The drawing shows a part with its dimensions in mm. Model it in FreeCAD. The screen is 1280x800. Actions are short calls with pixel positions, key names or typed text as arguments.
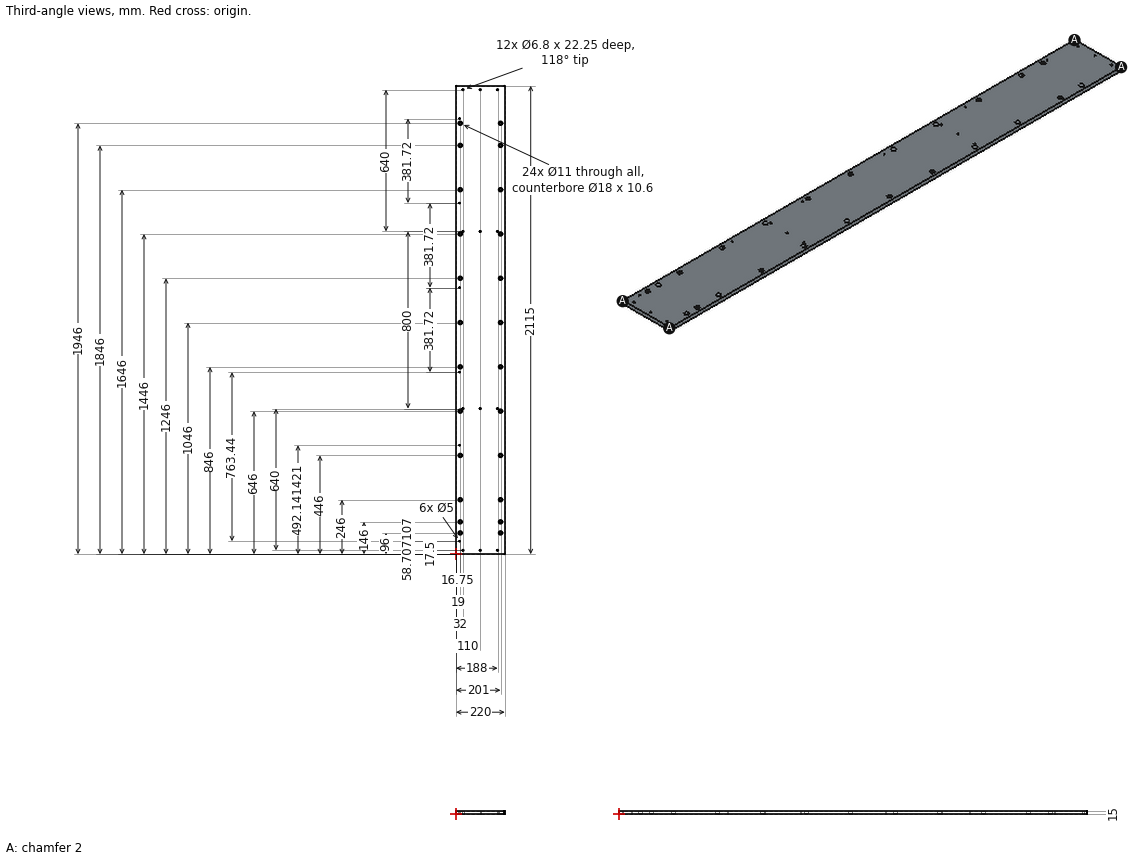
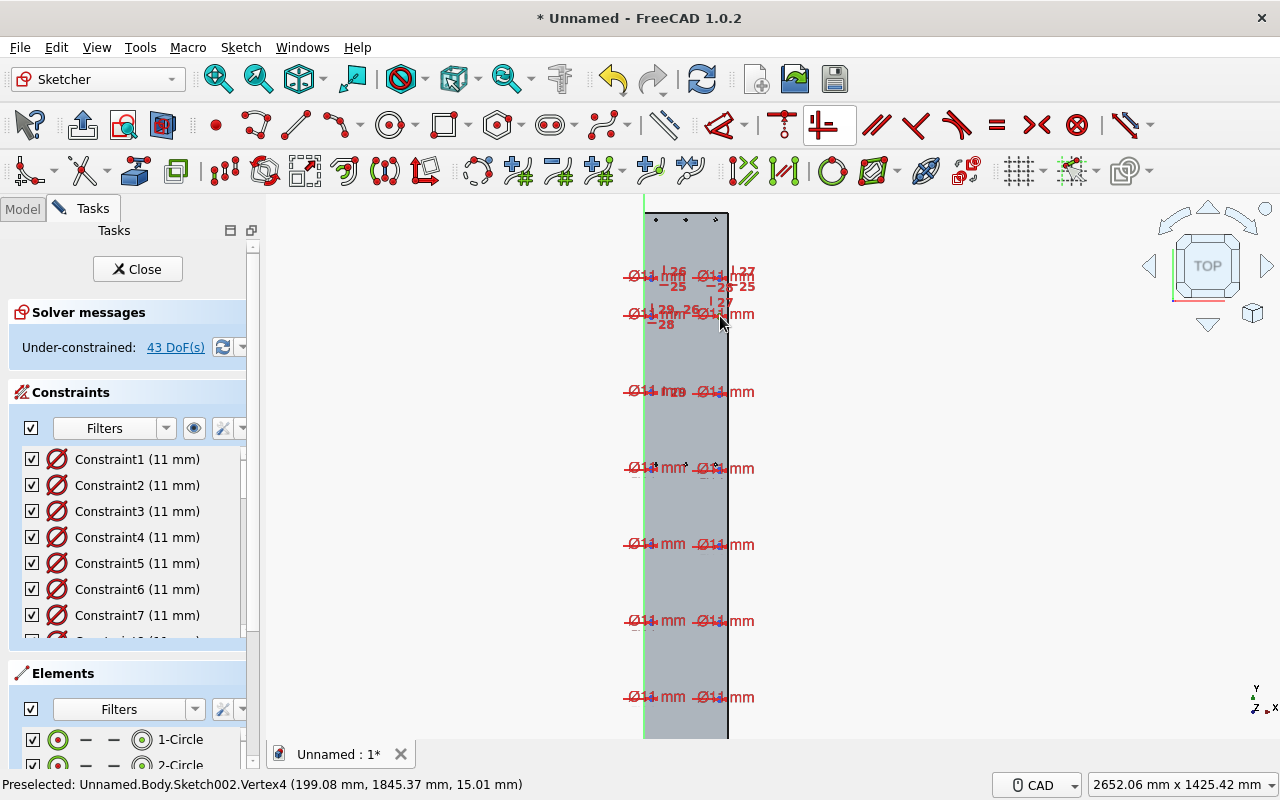
click(720, 394)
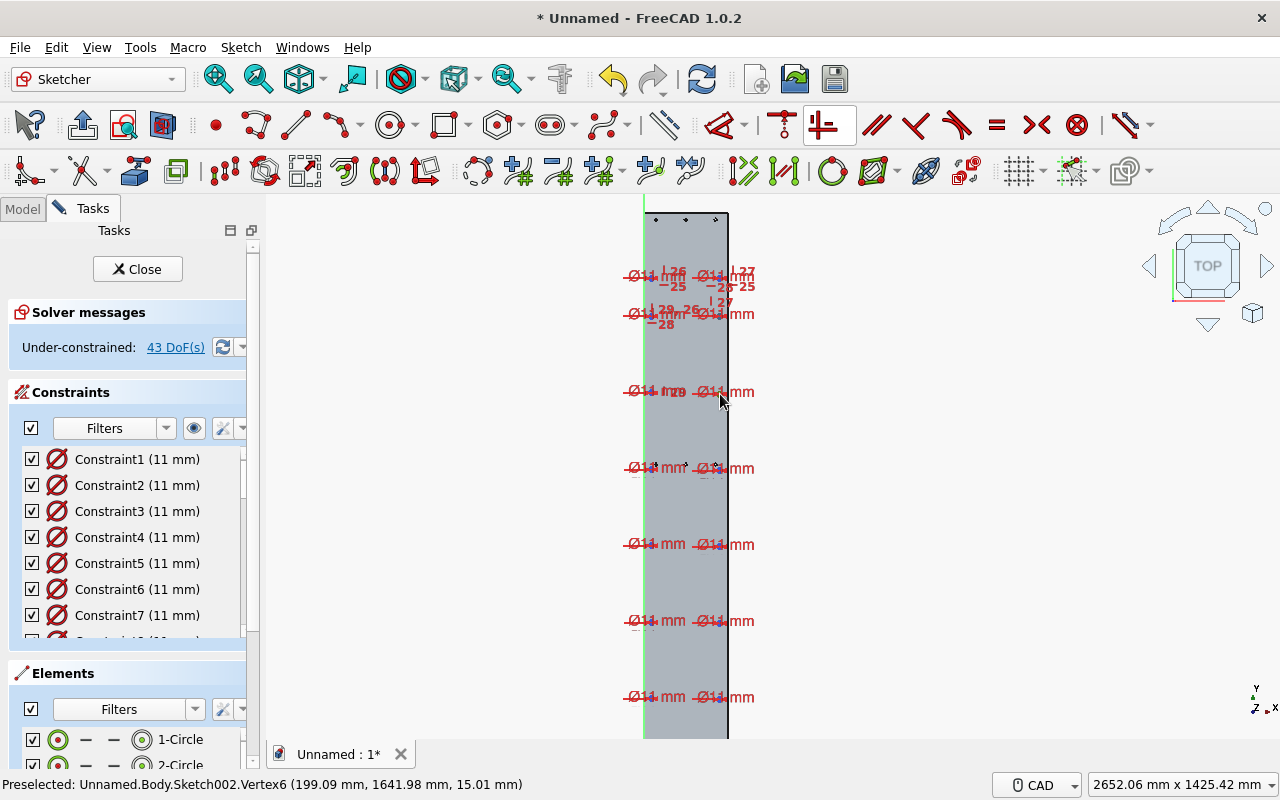
key(v)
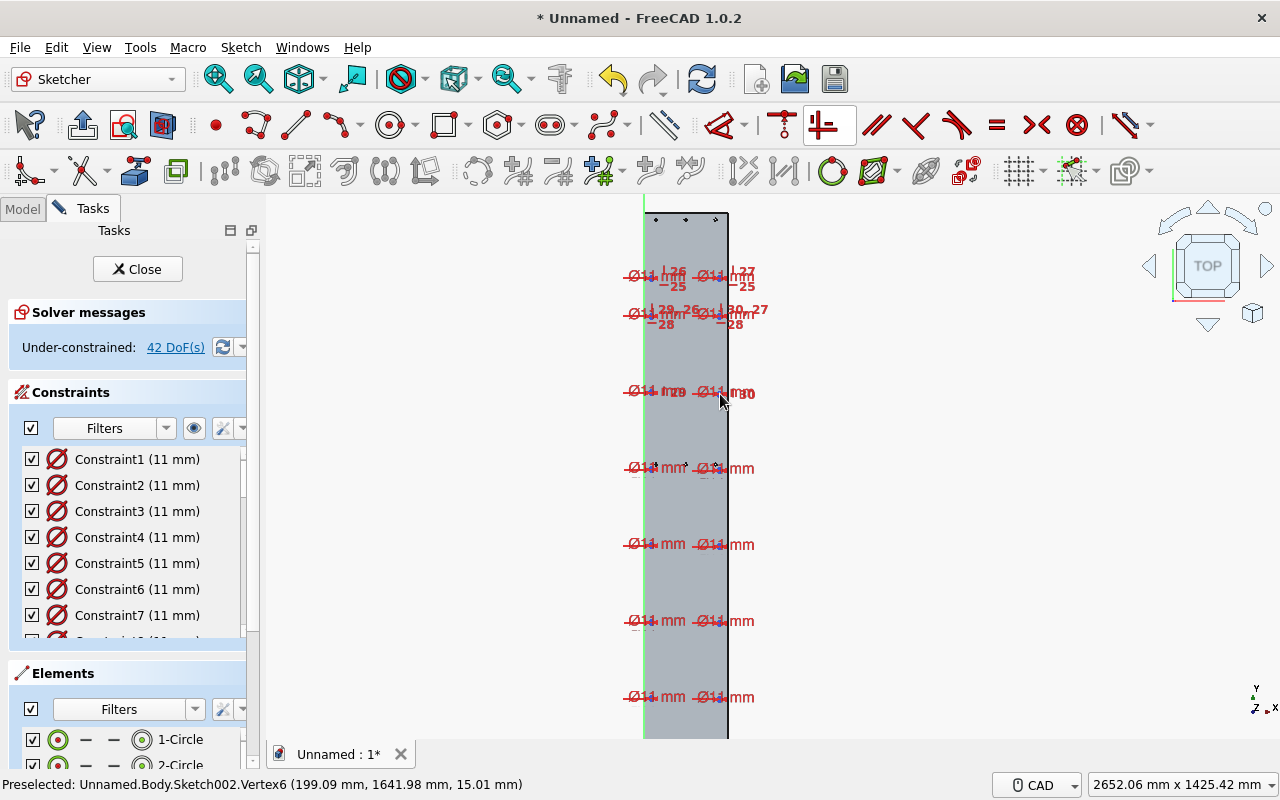
click(651, 393)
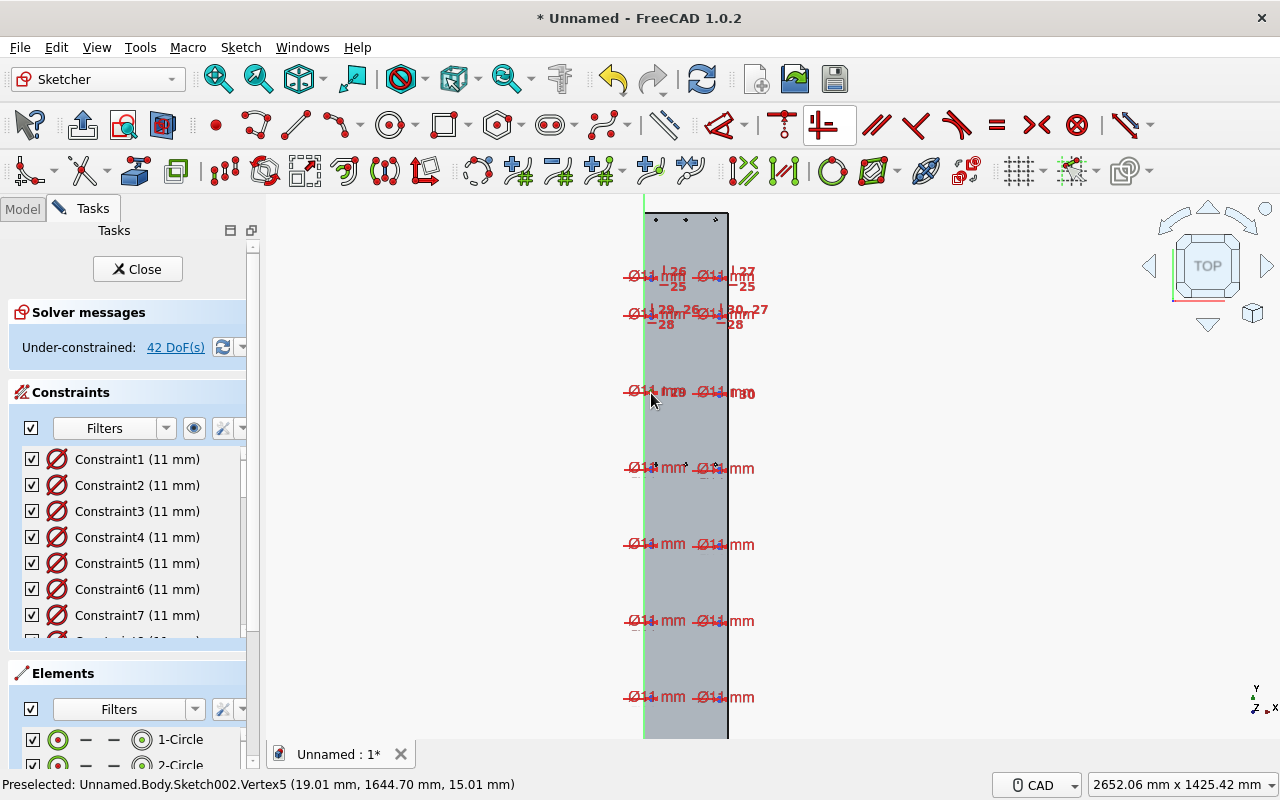
click(720, 394)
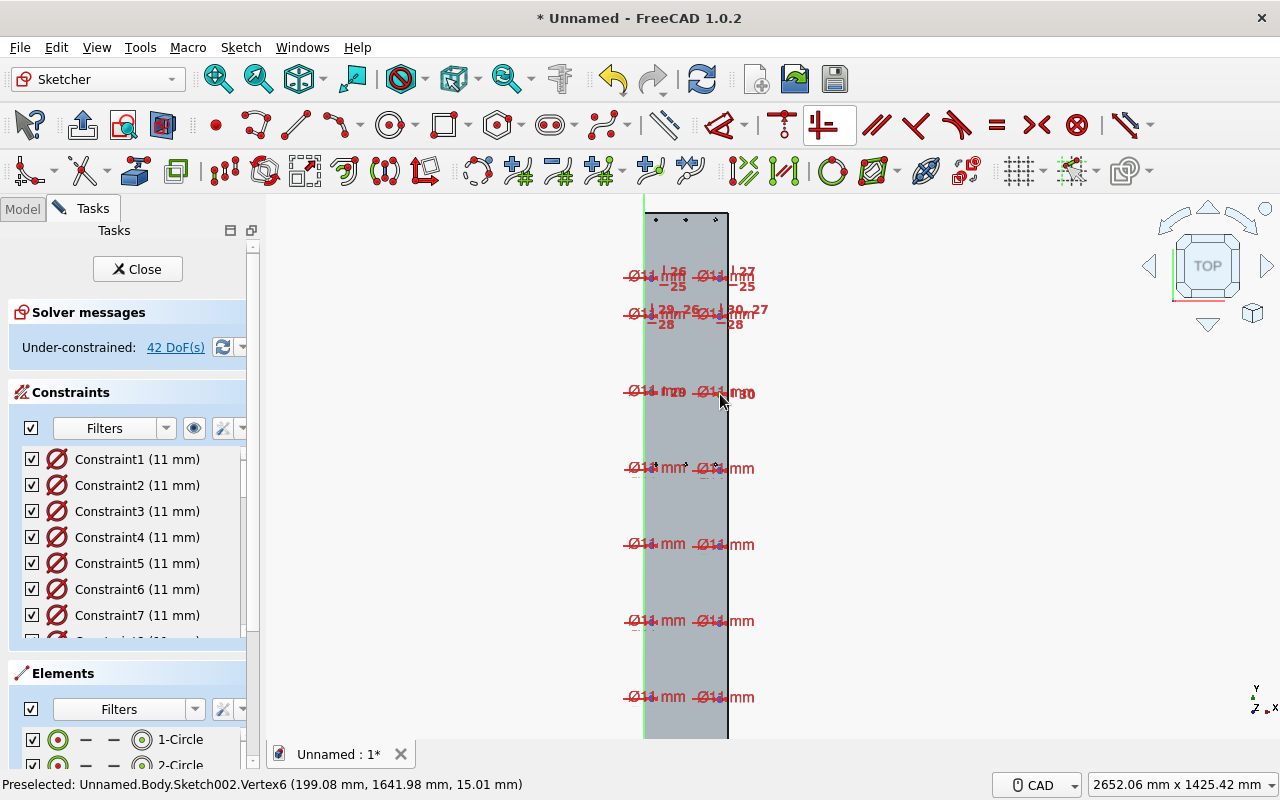
click(850, 126)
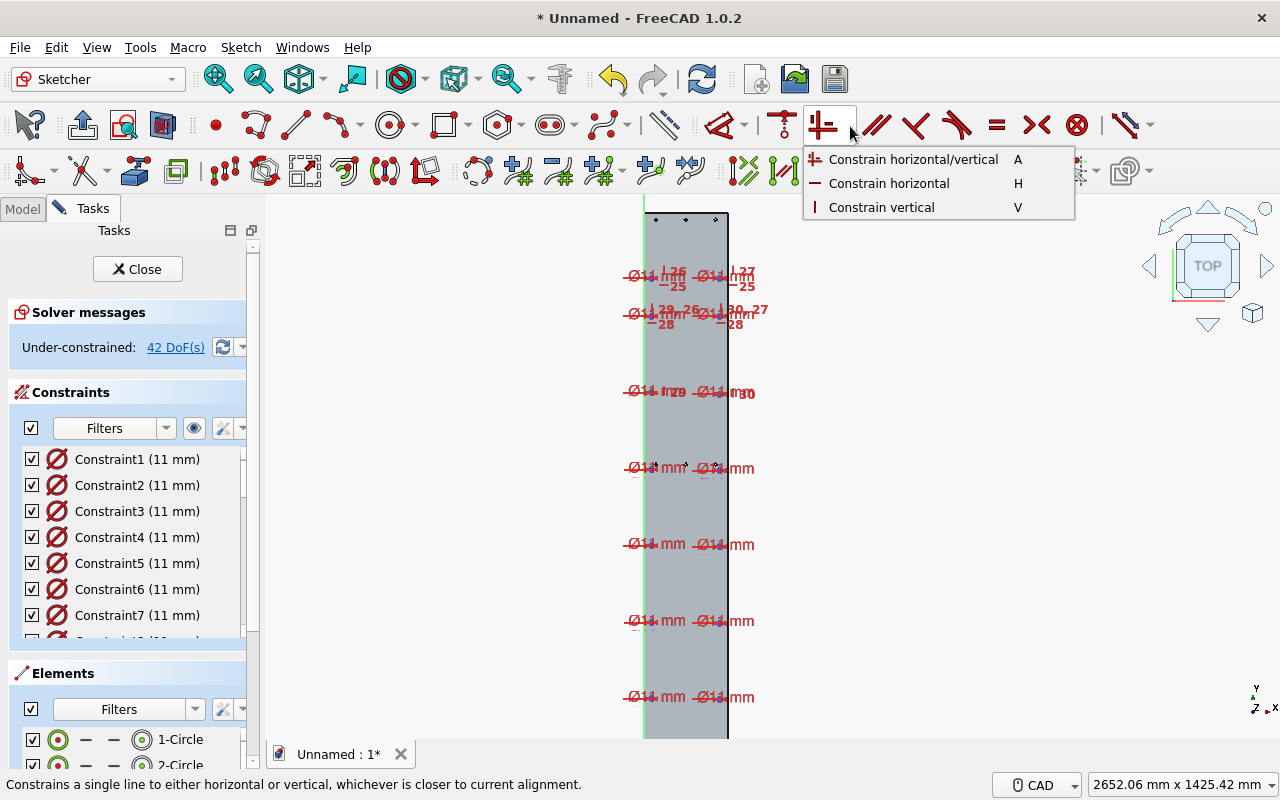
click(939, 183)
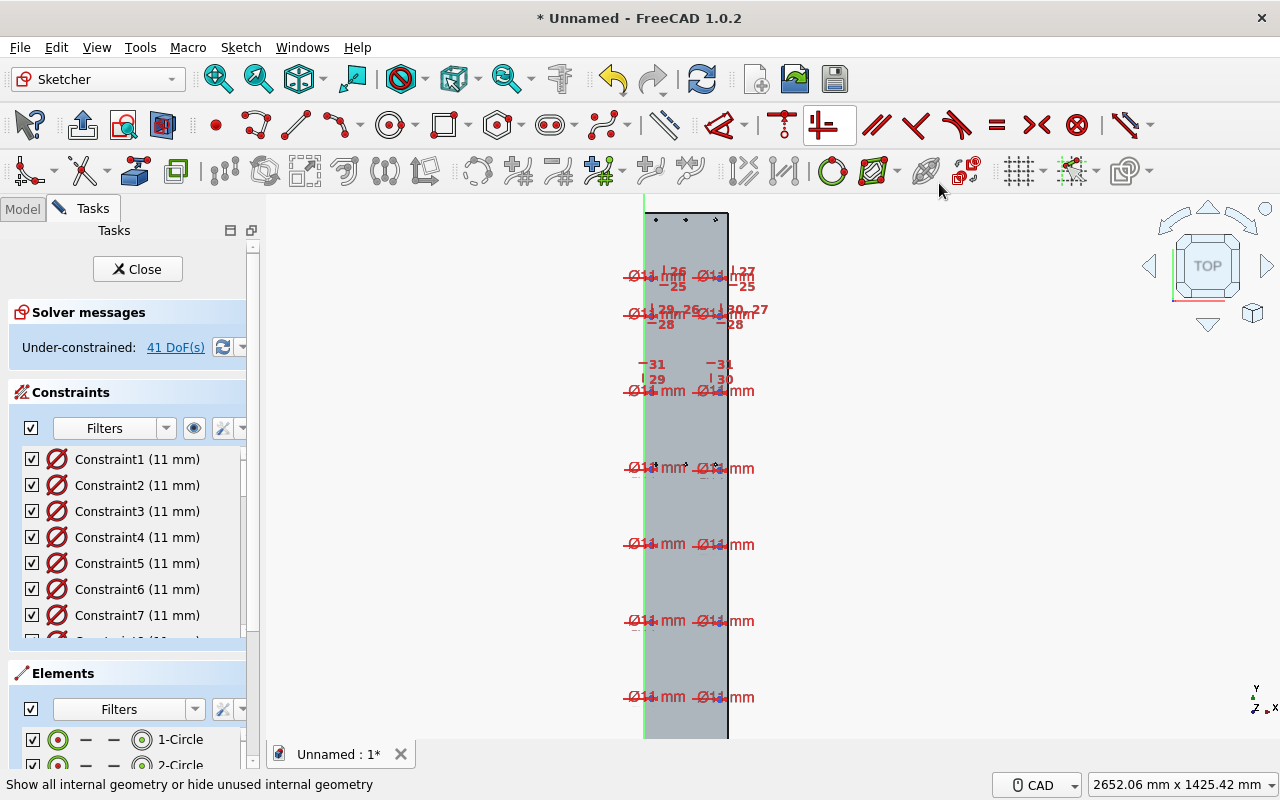
click(651, 393)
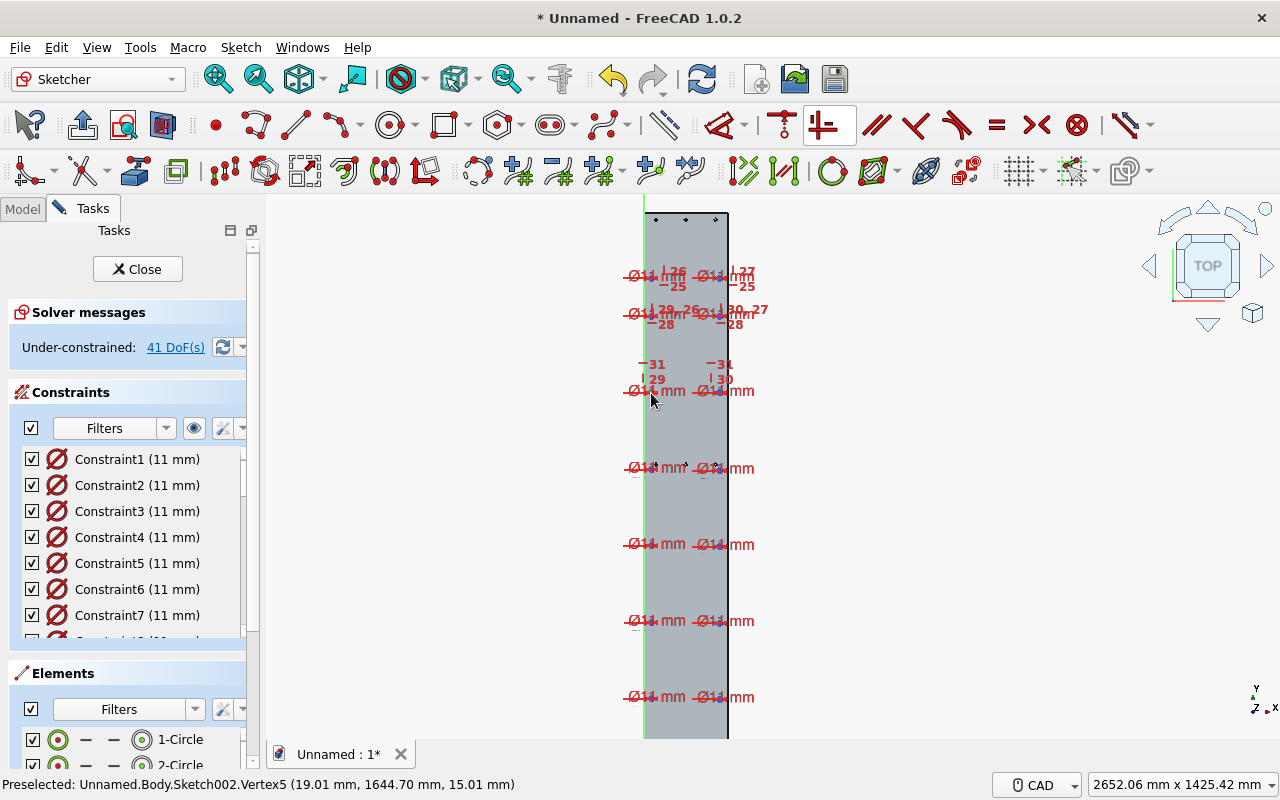
click(651, 470)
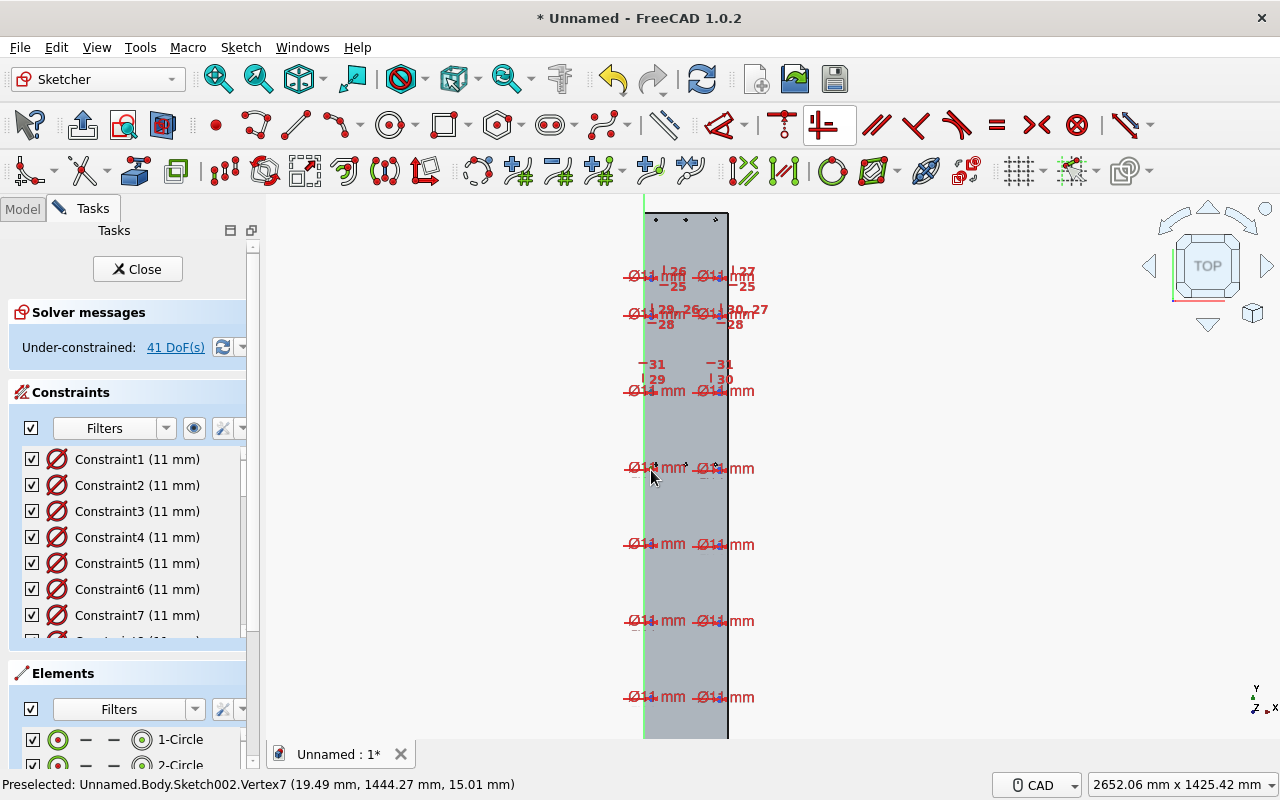
click(850, 126)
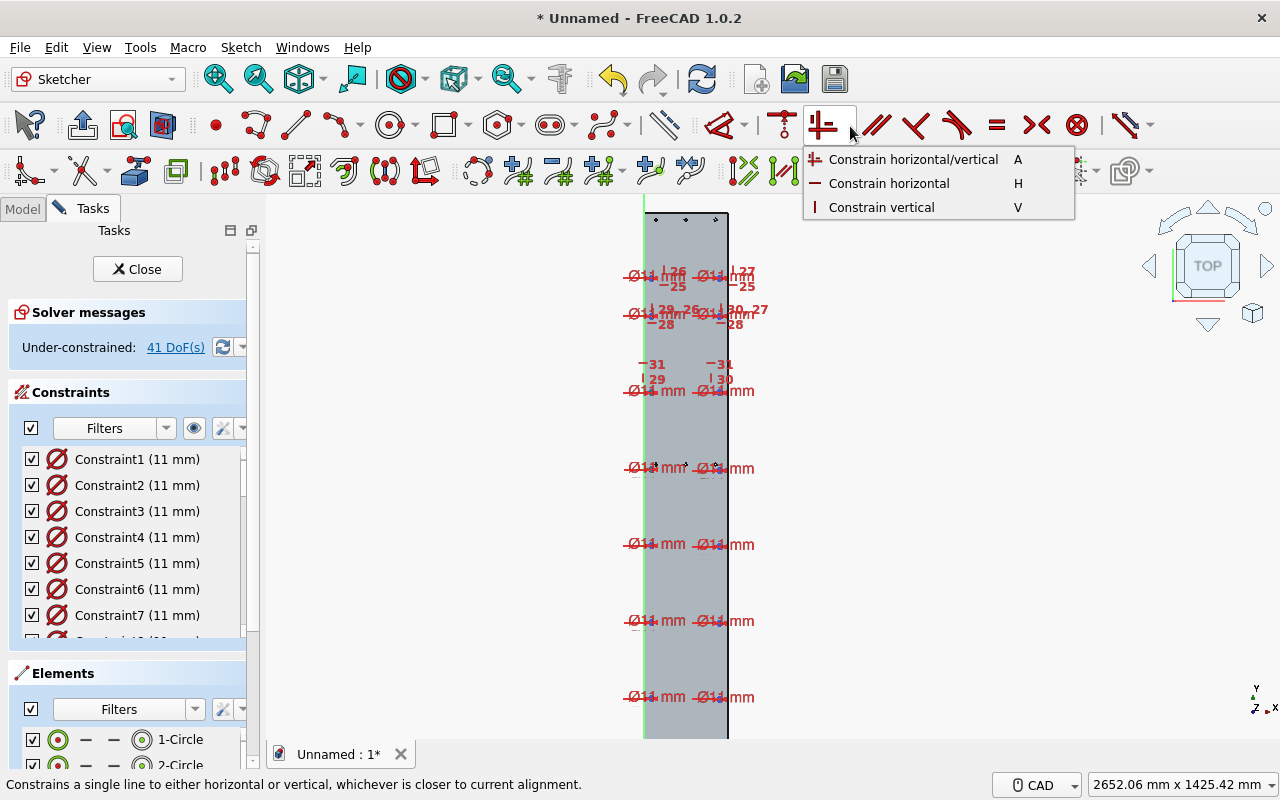
click(939, 207)